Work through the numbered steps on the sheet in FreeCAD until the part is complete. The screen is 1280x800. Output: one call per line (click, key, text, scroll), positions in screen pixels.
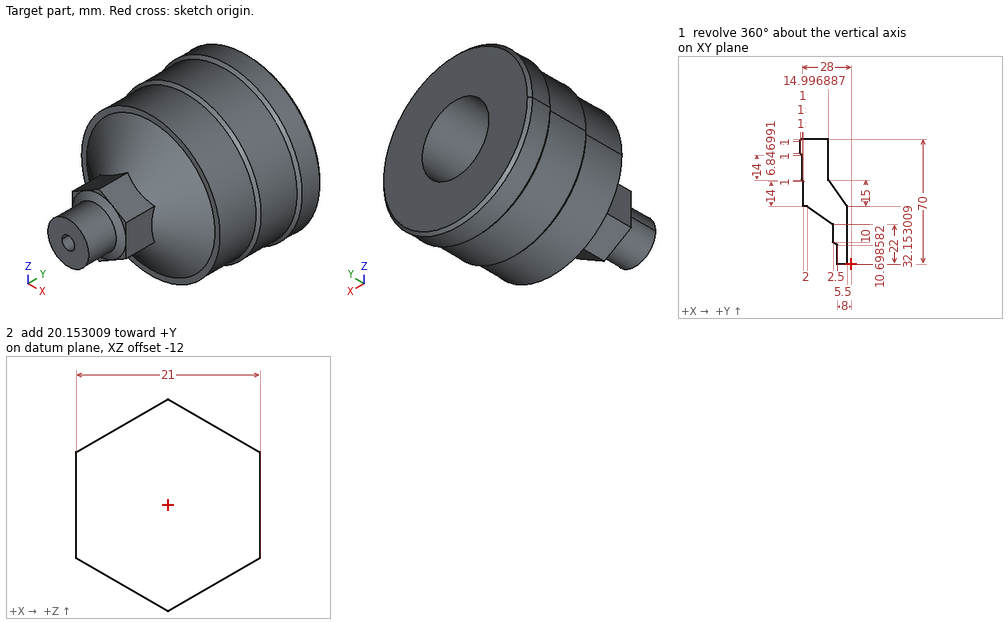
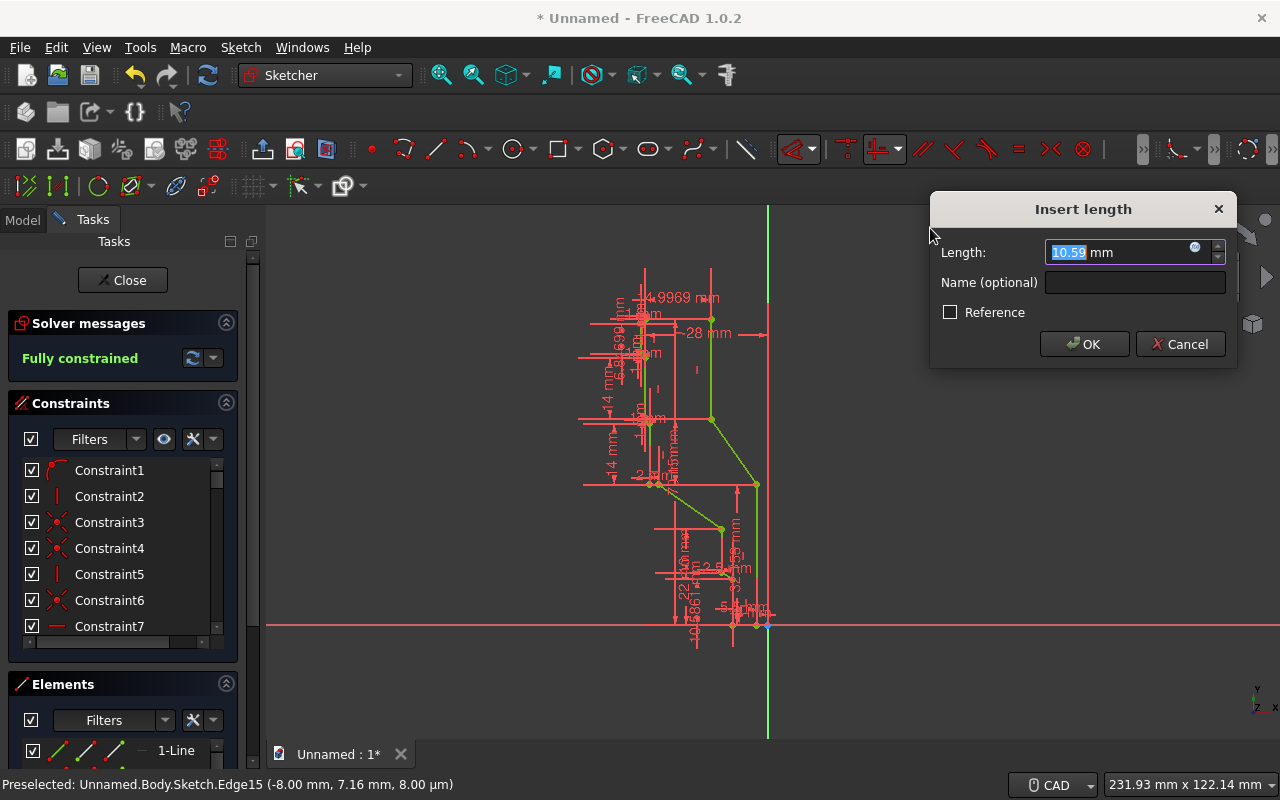
text(10.698582)
key(Return)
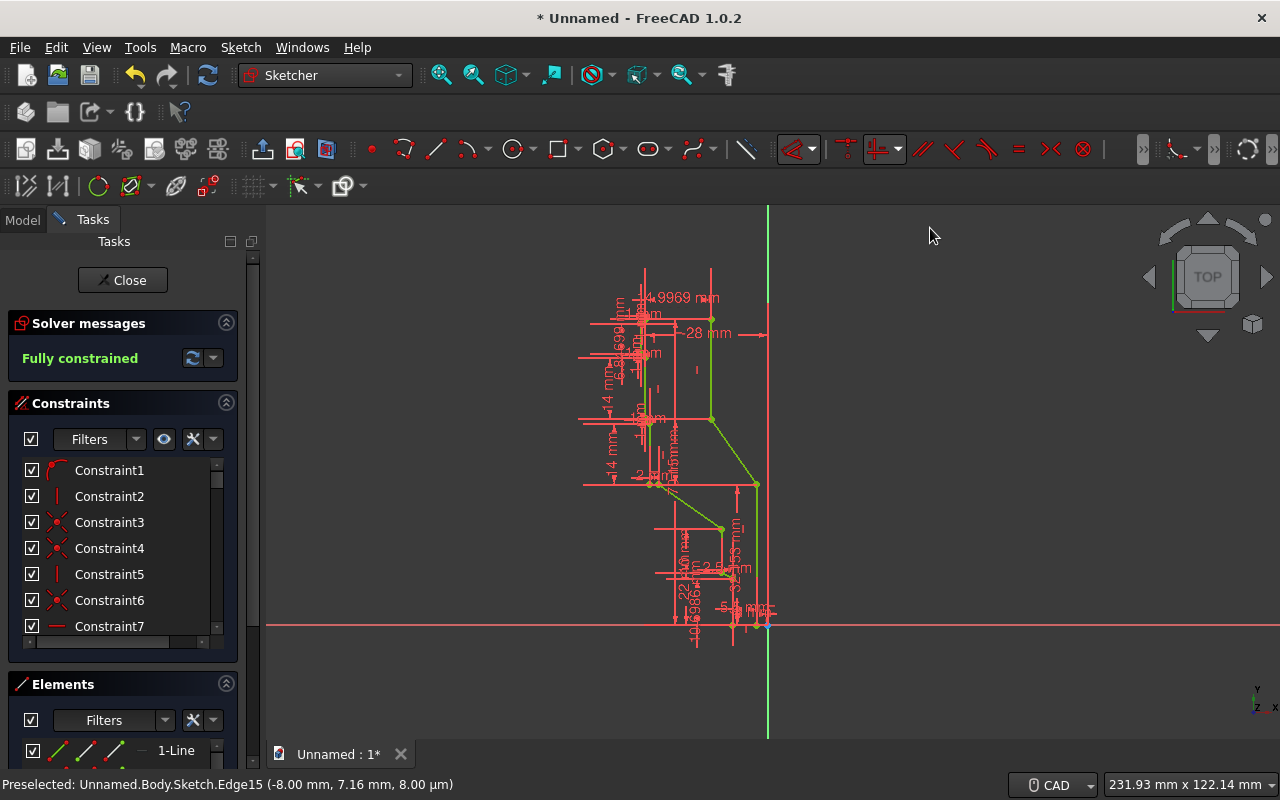
click(123, 280)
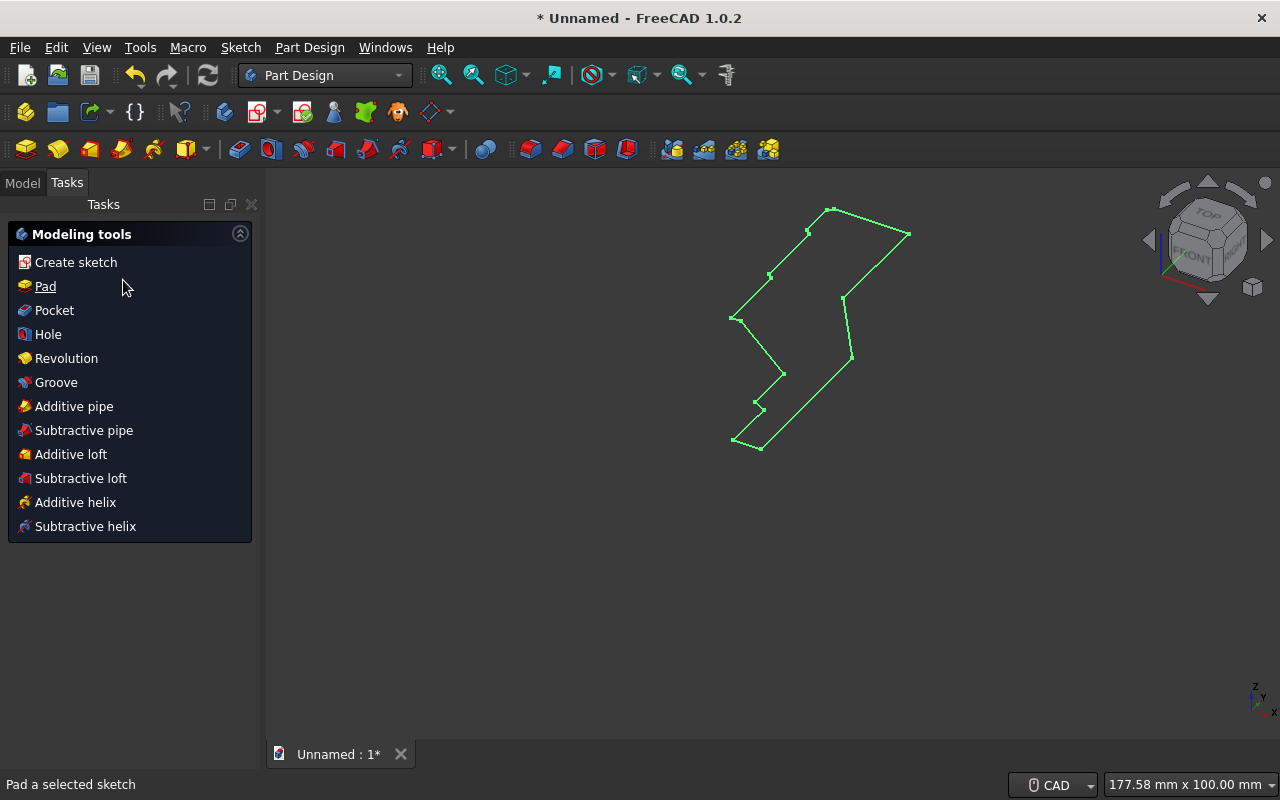
click(58, 150)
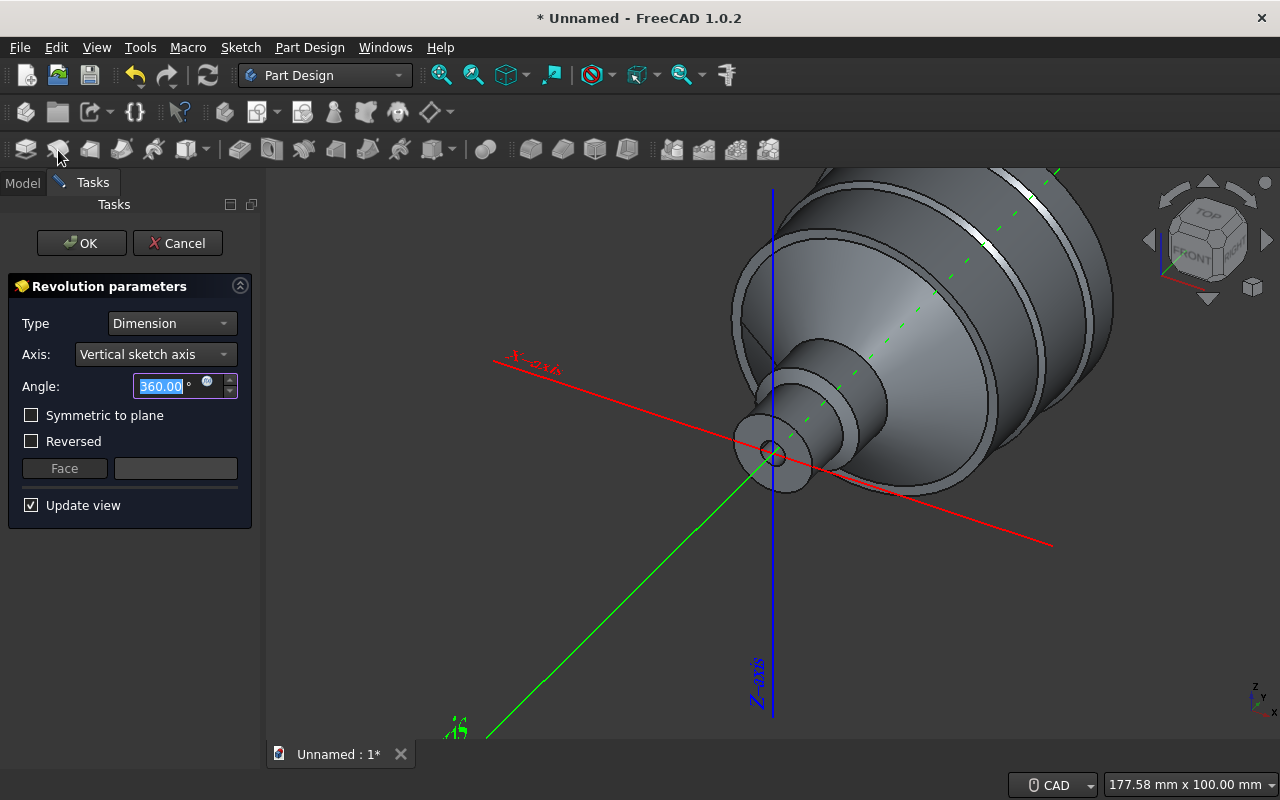
click(82, 243)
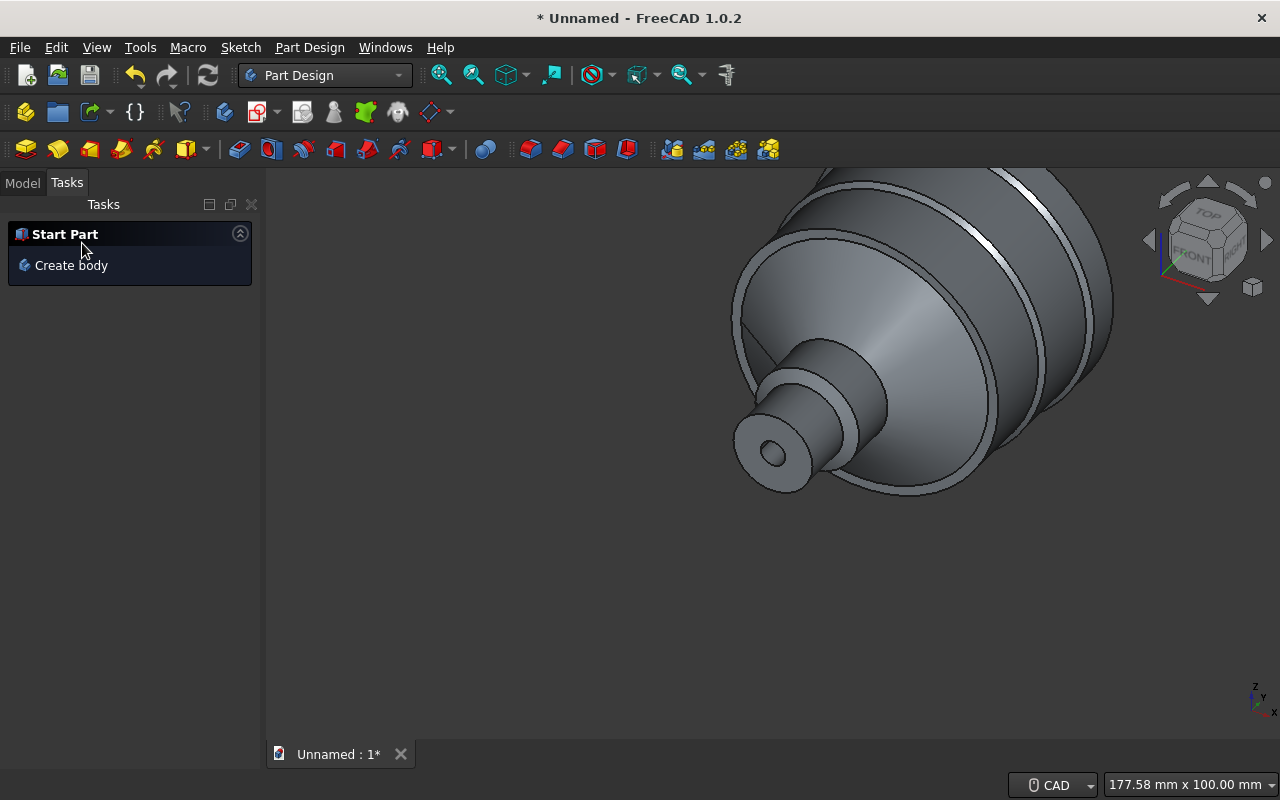
key(v)
key(f)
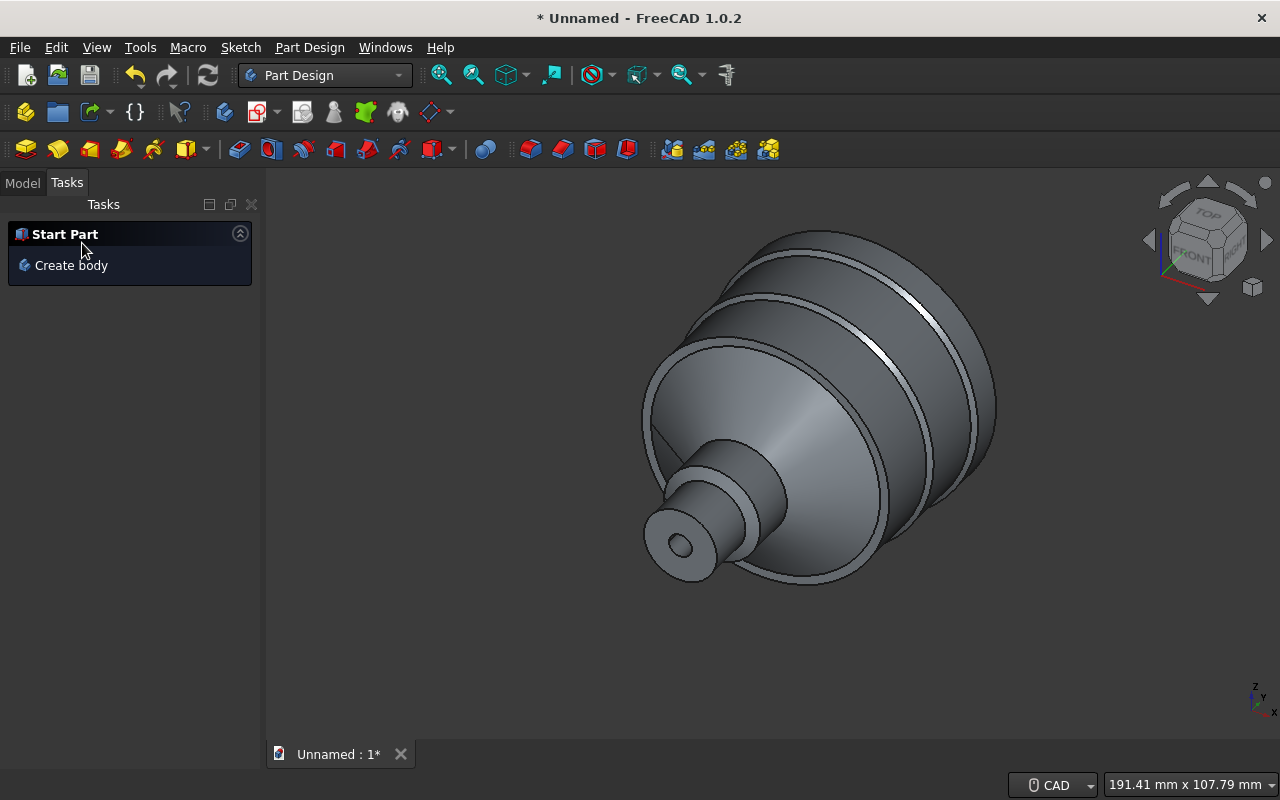
click(23, 182)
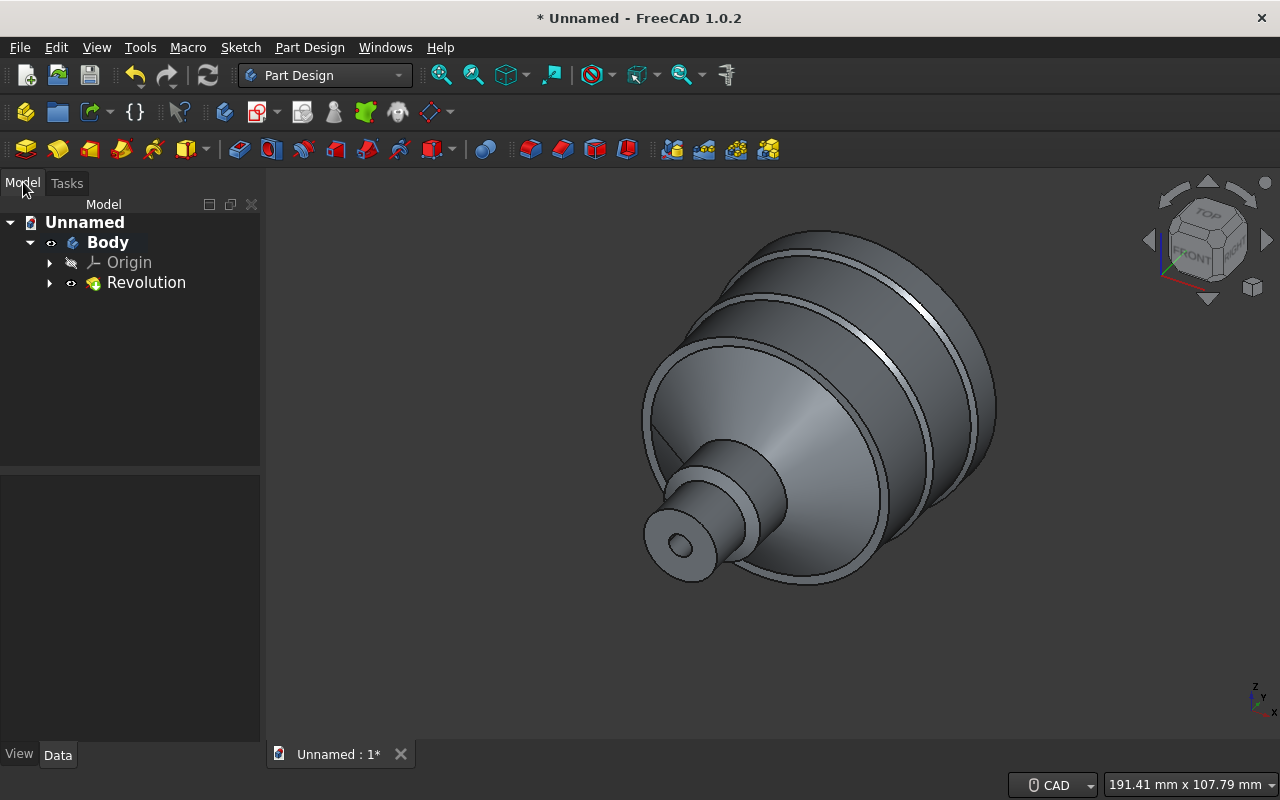
click(50, 263)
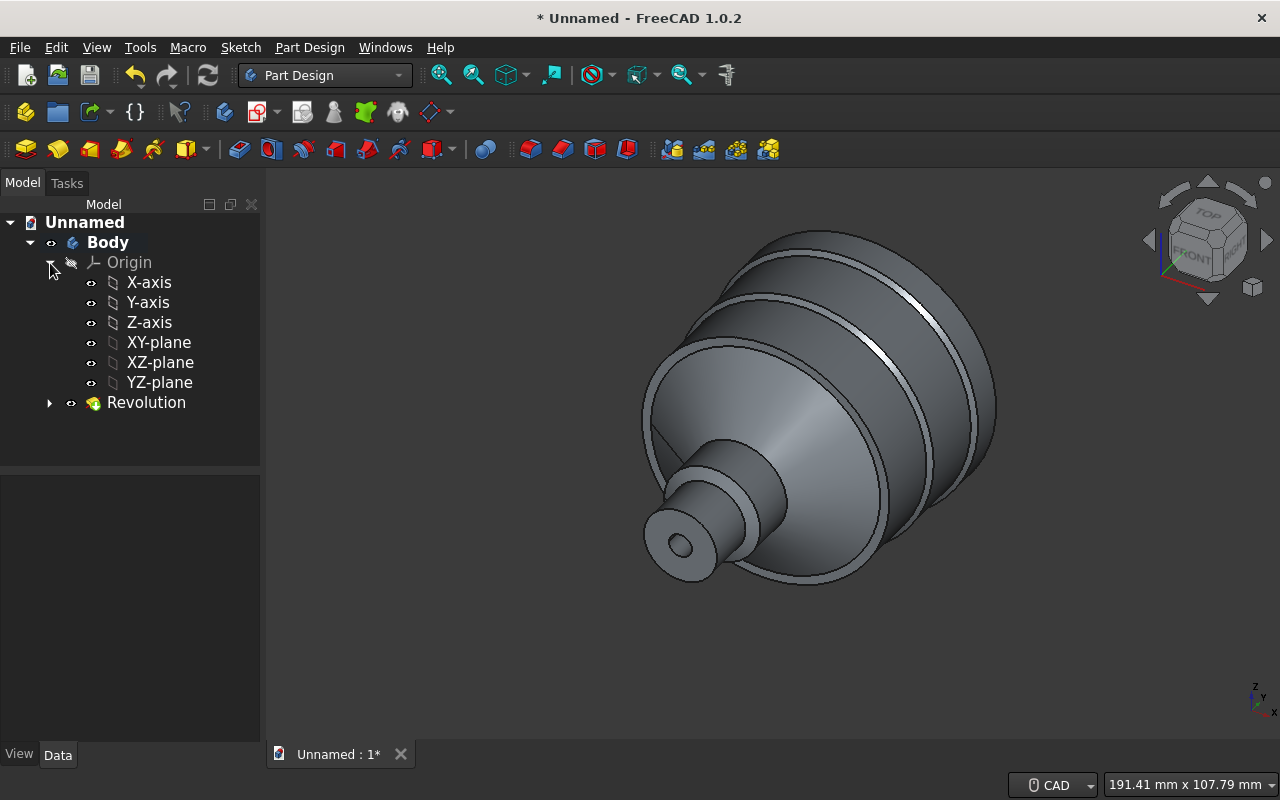
click(136, 363)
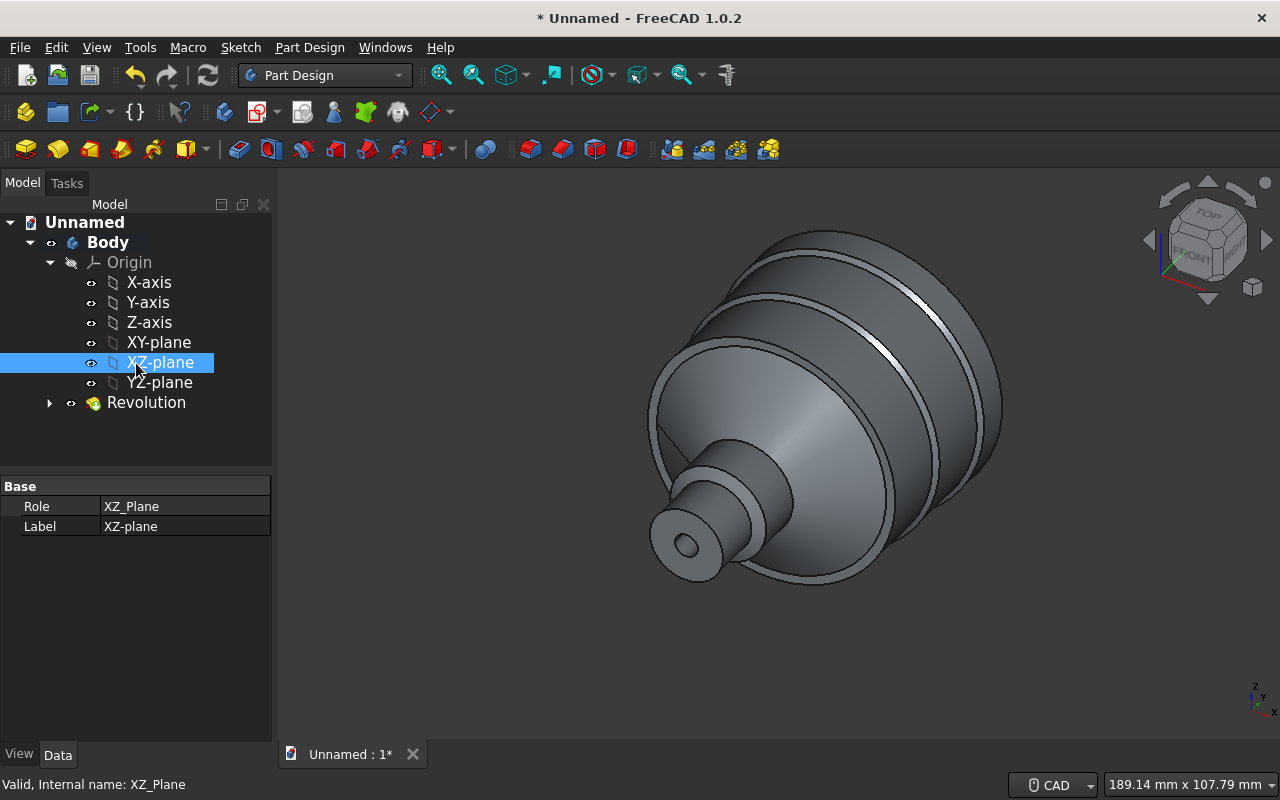
click(430, 112)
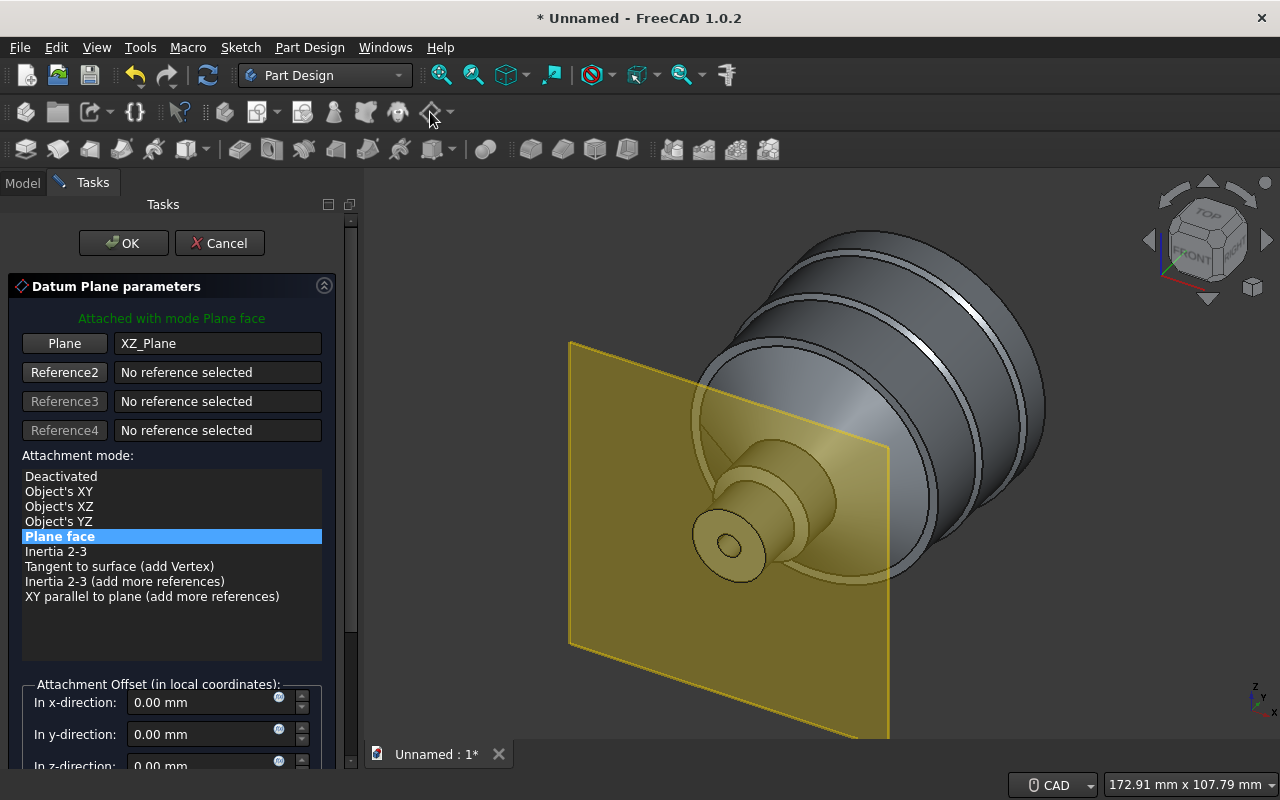
scroll(351, 491, down, 2)